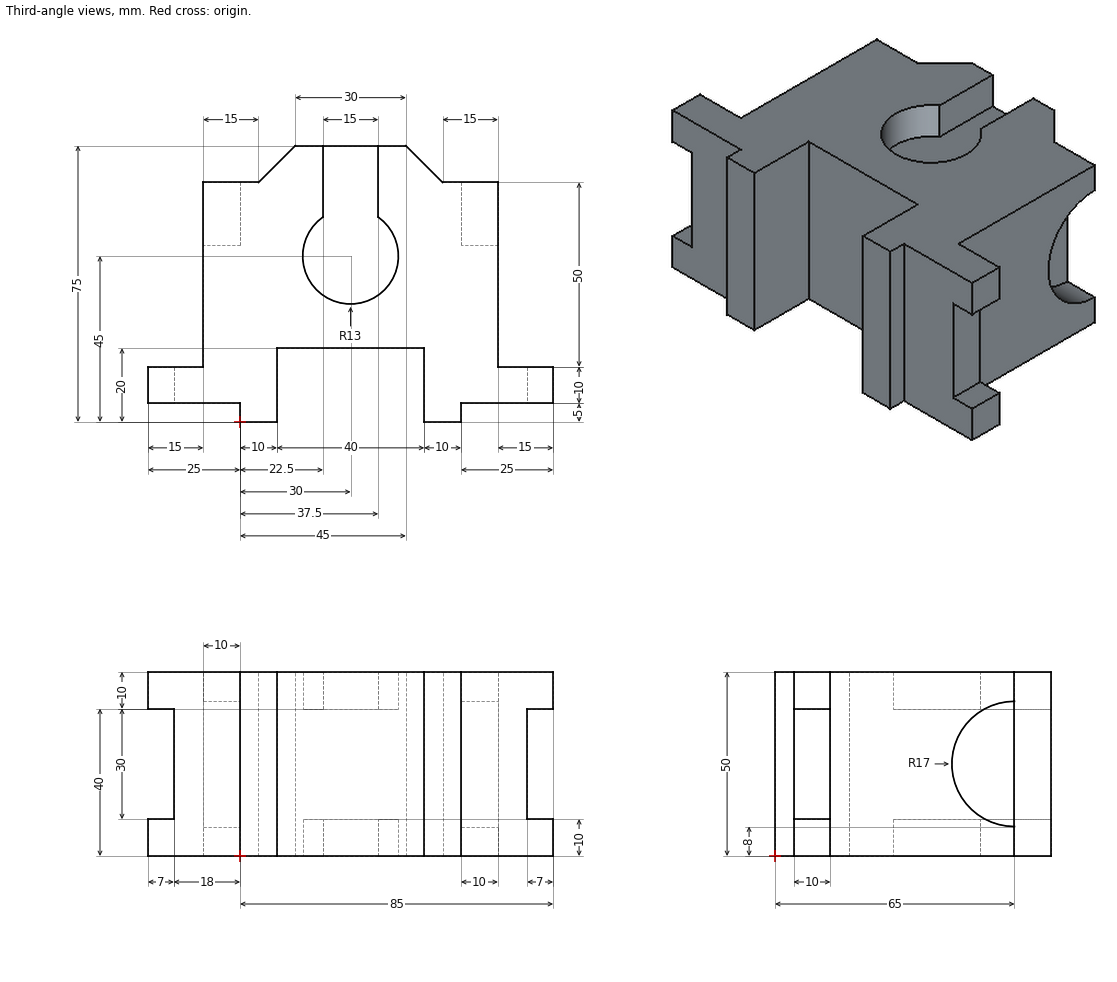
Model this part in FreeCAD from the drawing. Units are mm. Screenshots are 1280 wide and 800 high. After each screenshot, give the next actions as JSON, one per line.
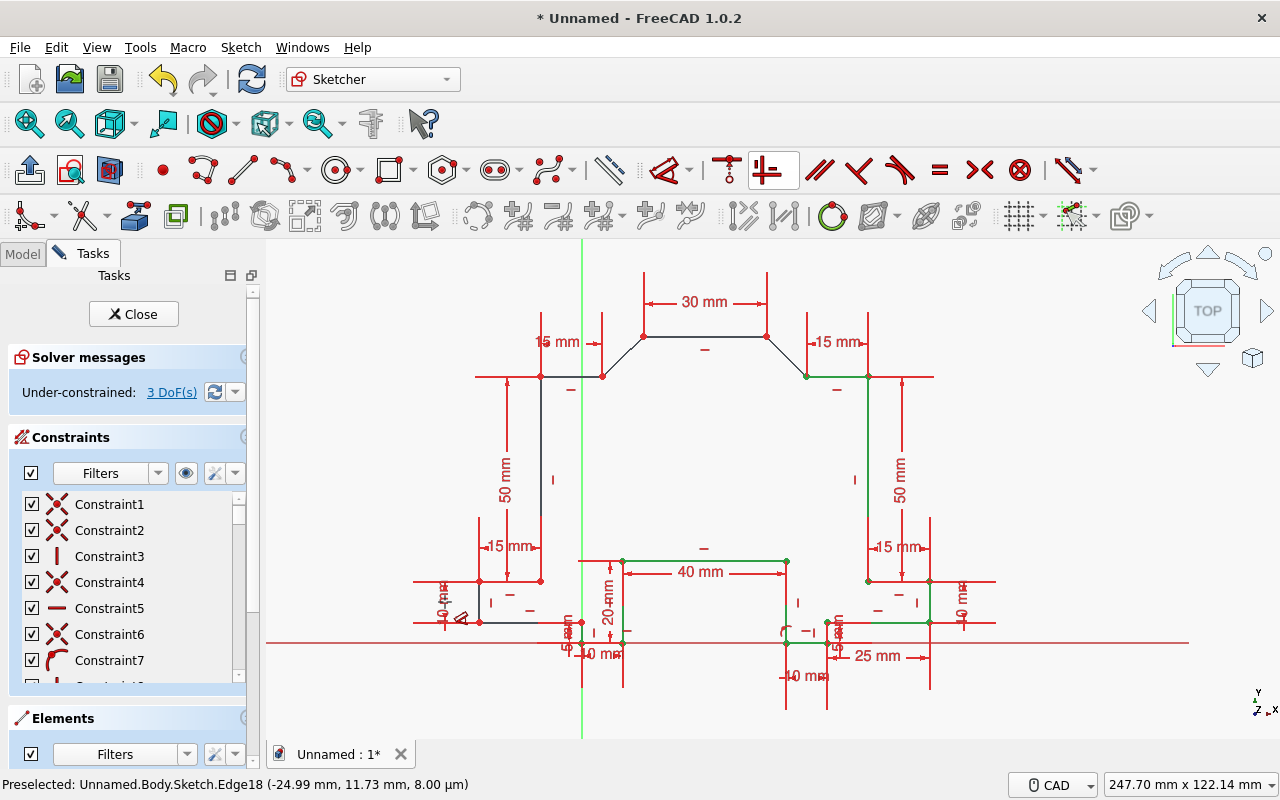
{"action": "left_click", "coordinate": [510, 623]}
{"action": "left_click", "coordinate": [531, 657]}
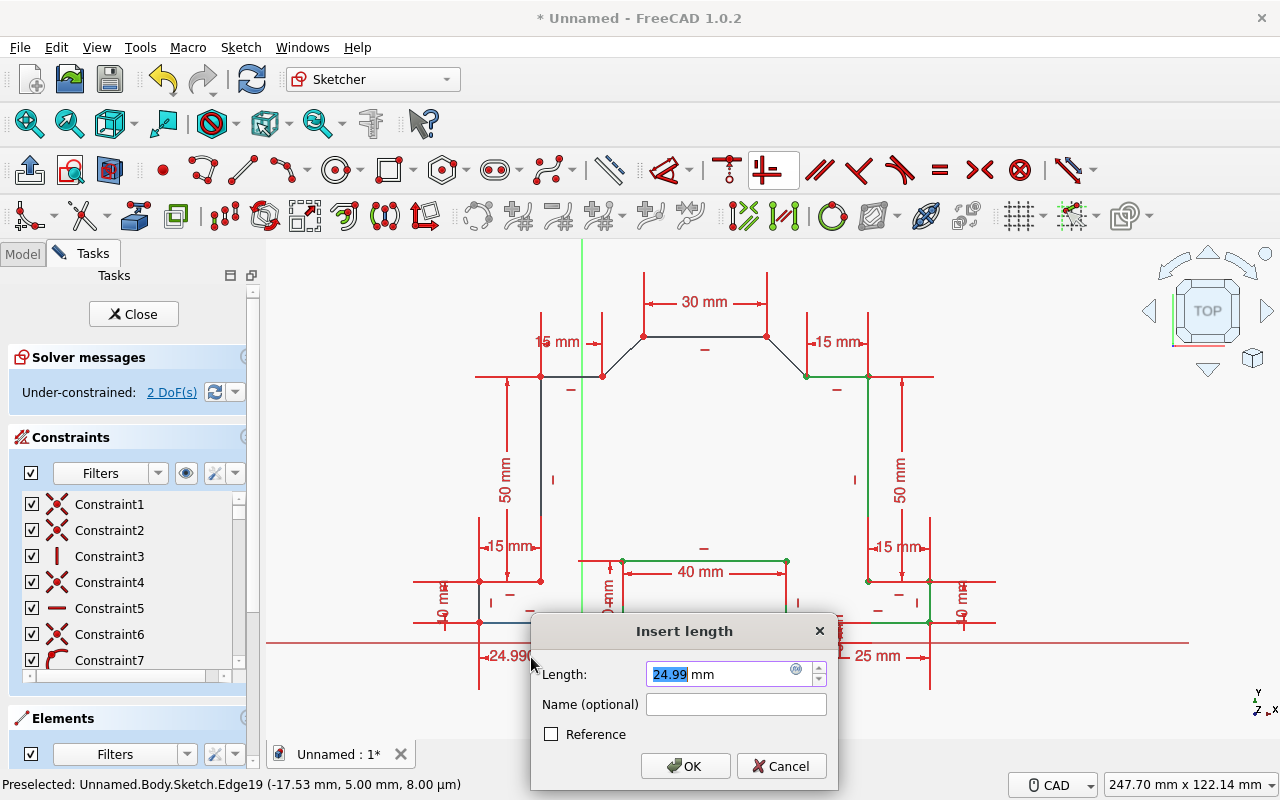
{"action": "type", "text": "25"}
{"action": "key", "text": "Return"}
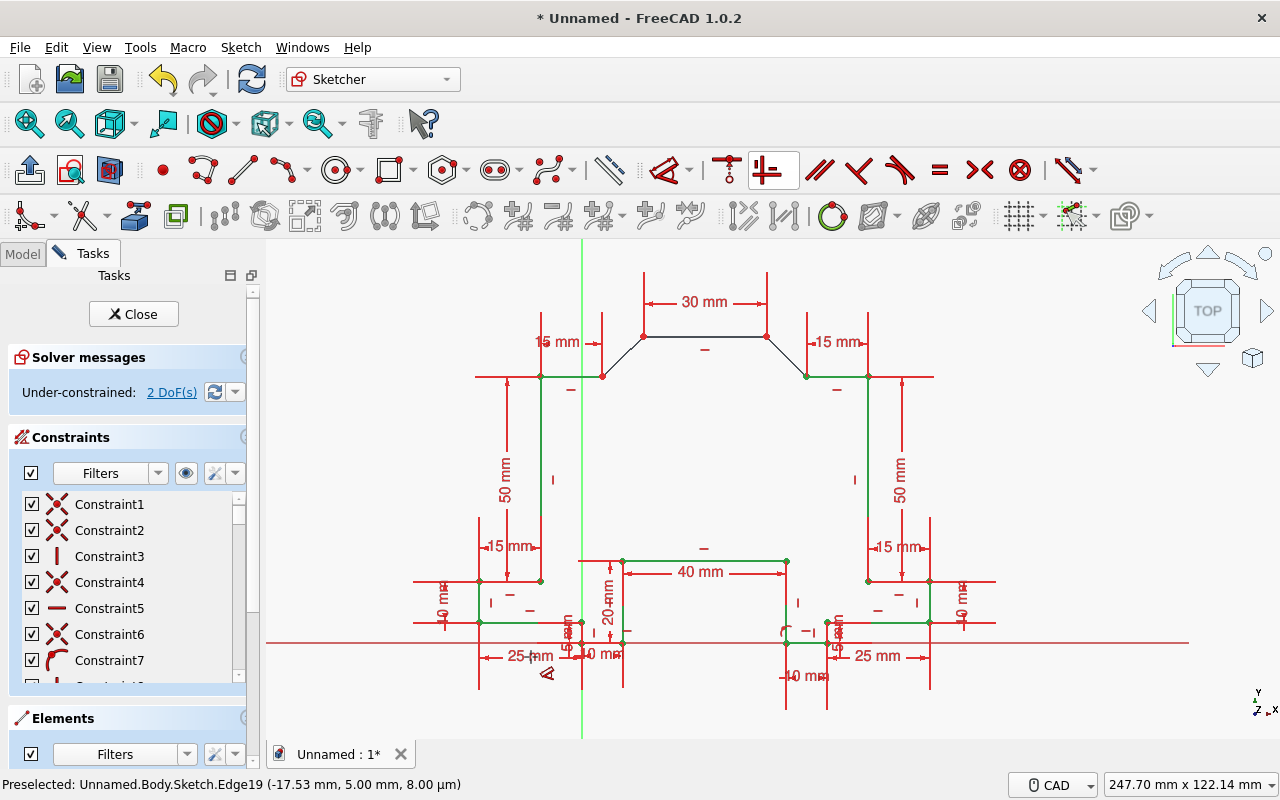
{"action": "left_click", "coordinate": [767, 337]}
{"action": "left_click", "coordinate": [674, 677]}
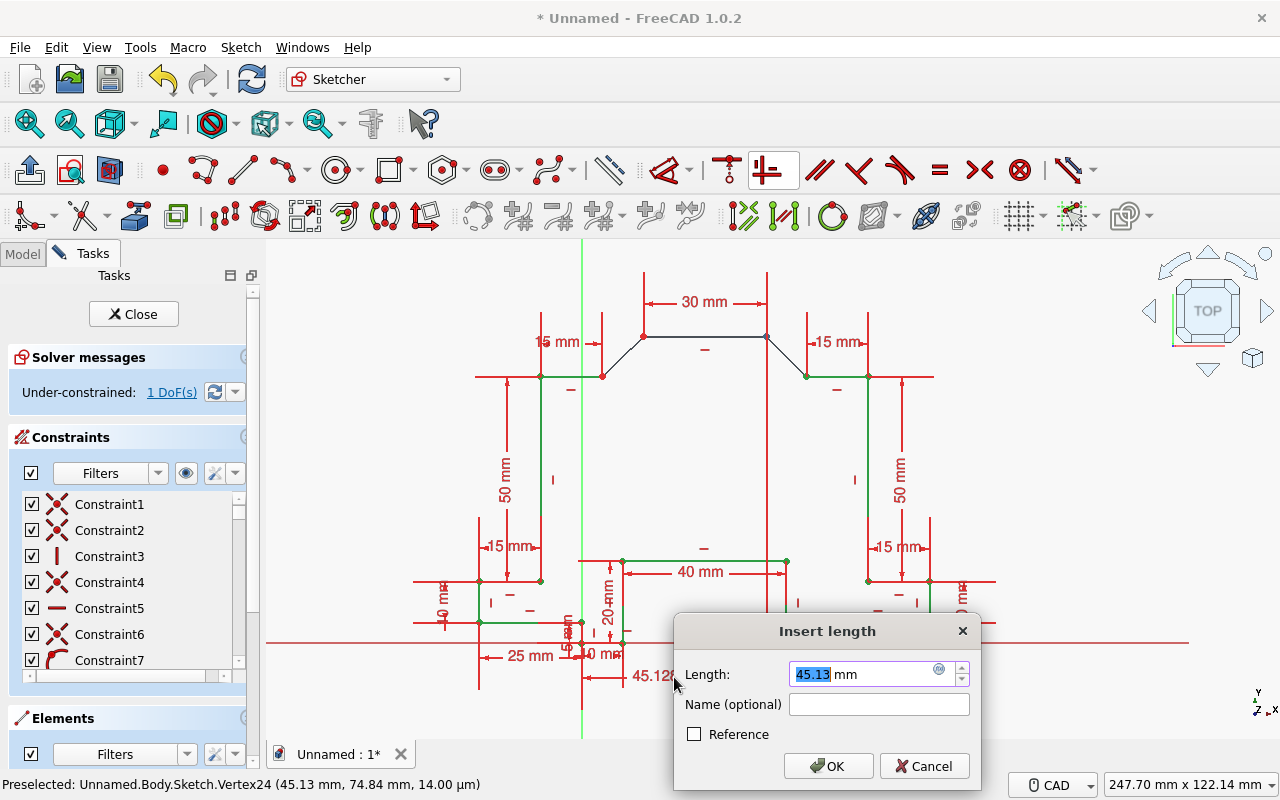
{"action": "type", "text": "45"}
{"action": "key", "text": "Return"}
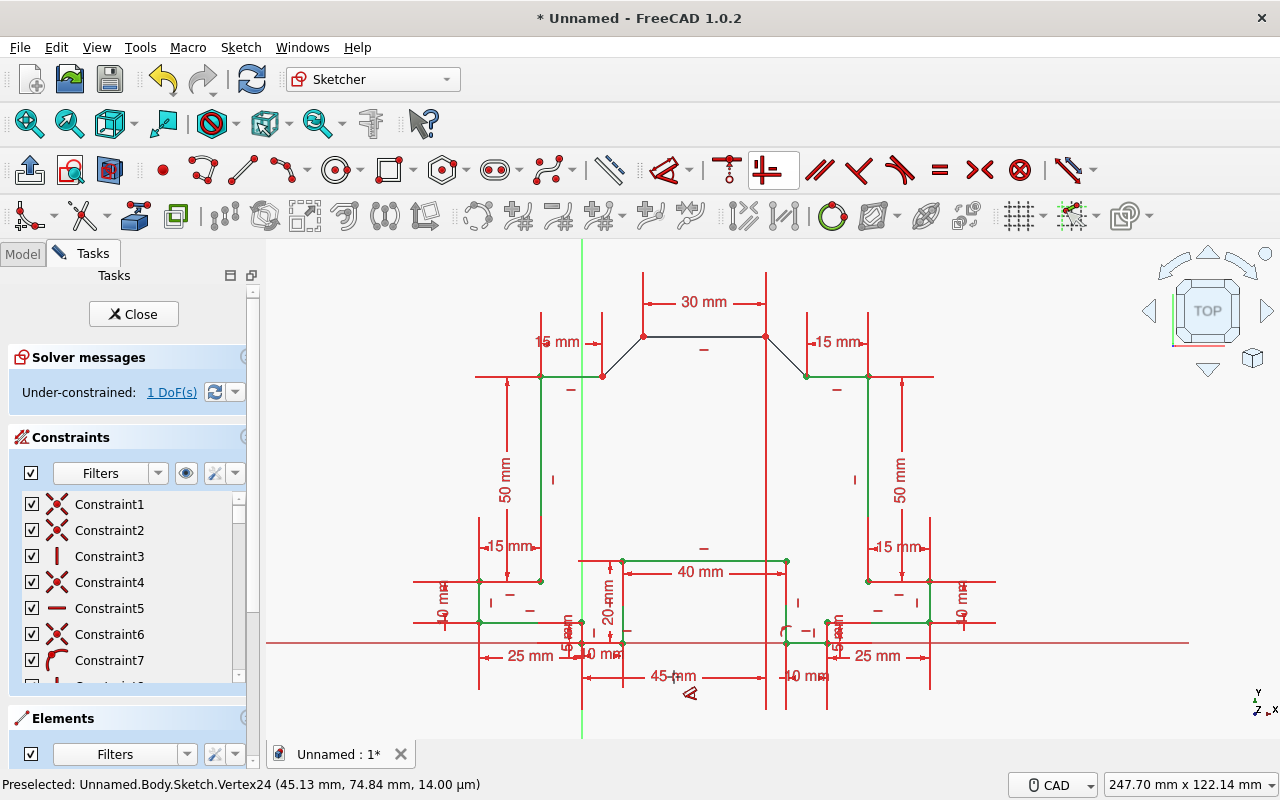
{"action": "left_click", "coordinate": [766, 337]}
{"action": "left_click", "coordinate": [800, 490]}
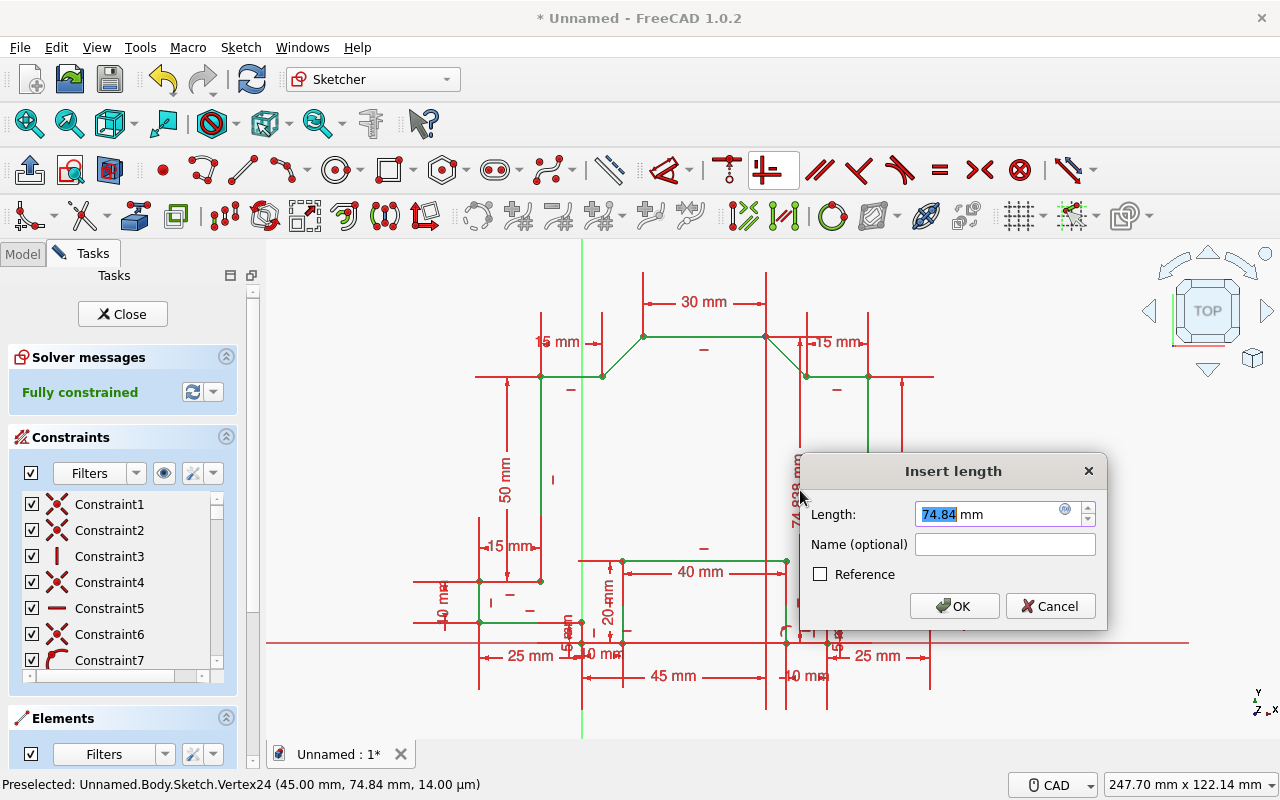
{"action": "type", "text": "75"}
{"action": "key", "text": "Return"}
{"action": "key", "text": "Escape"}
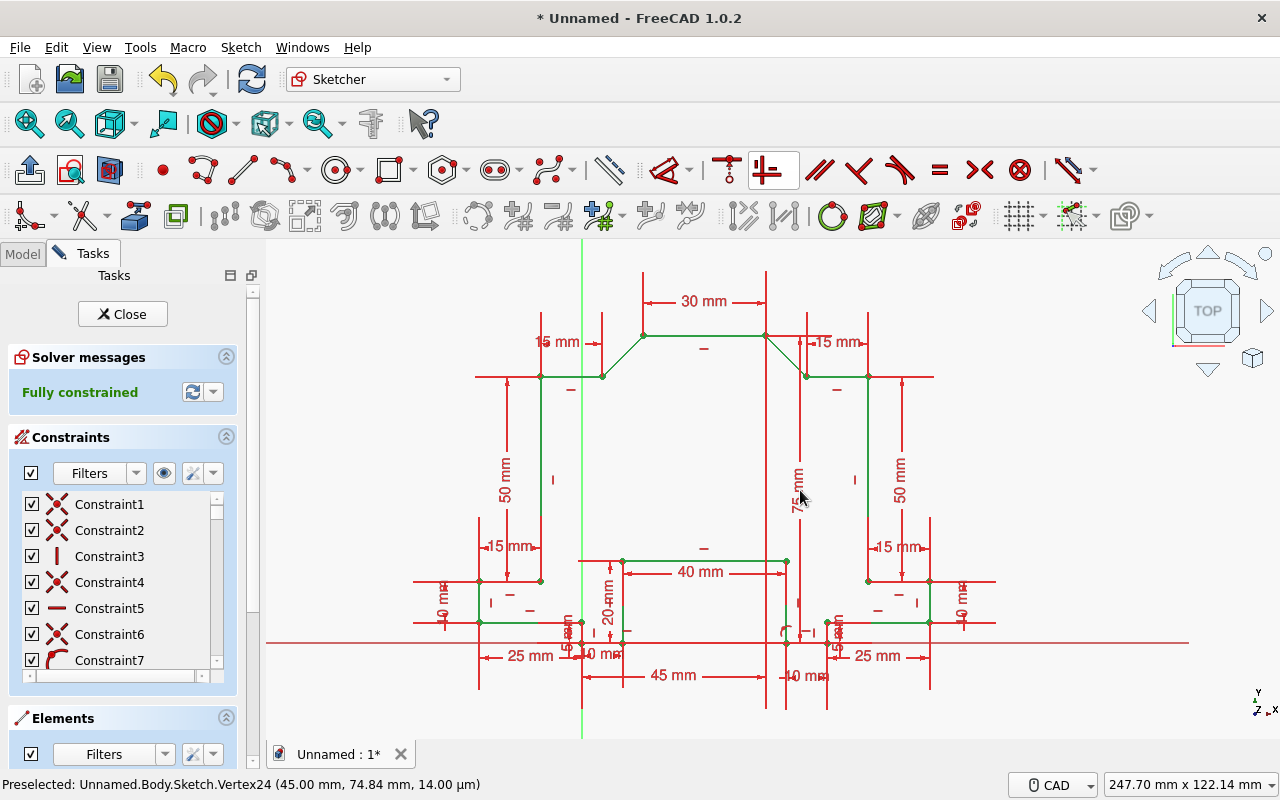
{"action": "left_click", "coordinate": [123, 314]}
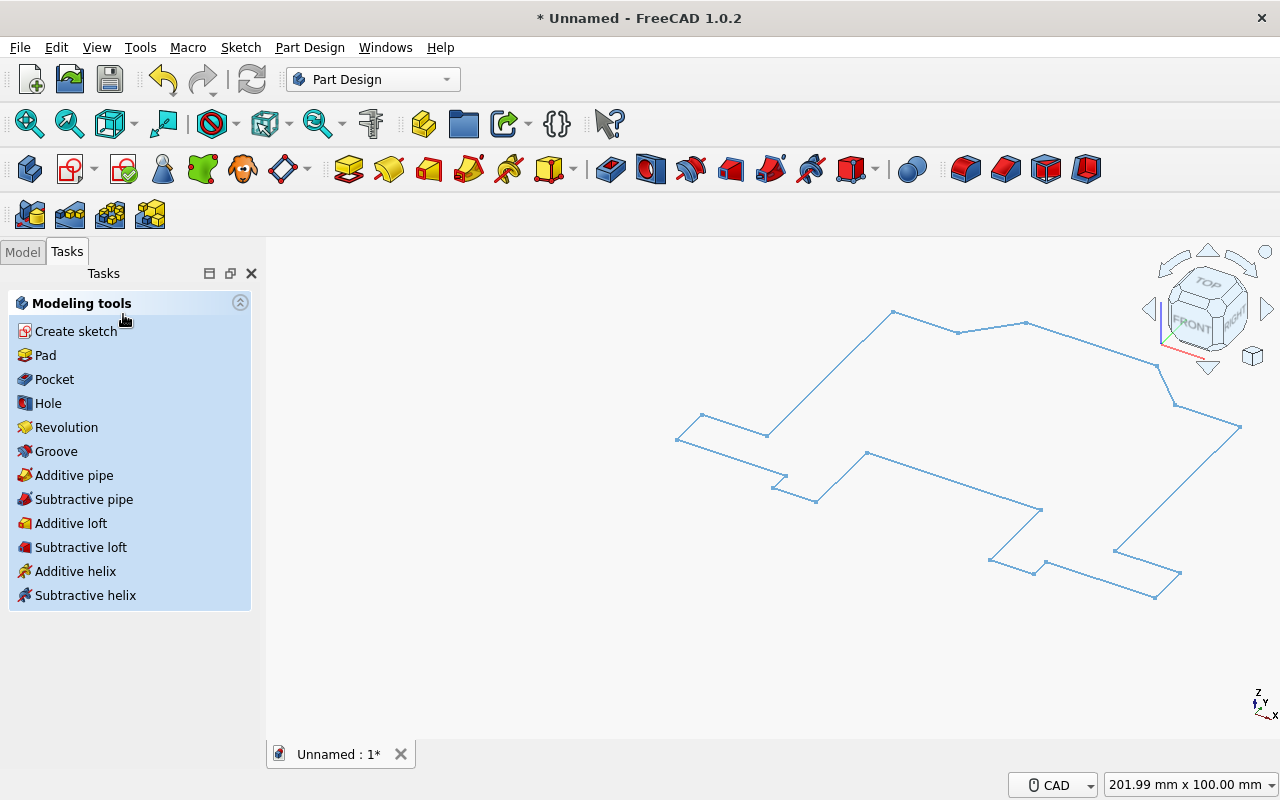
{"action": "left_click", "coordinate": [350, 170]}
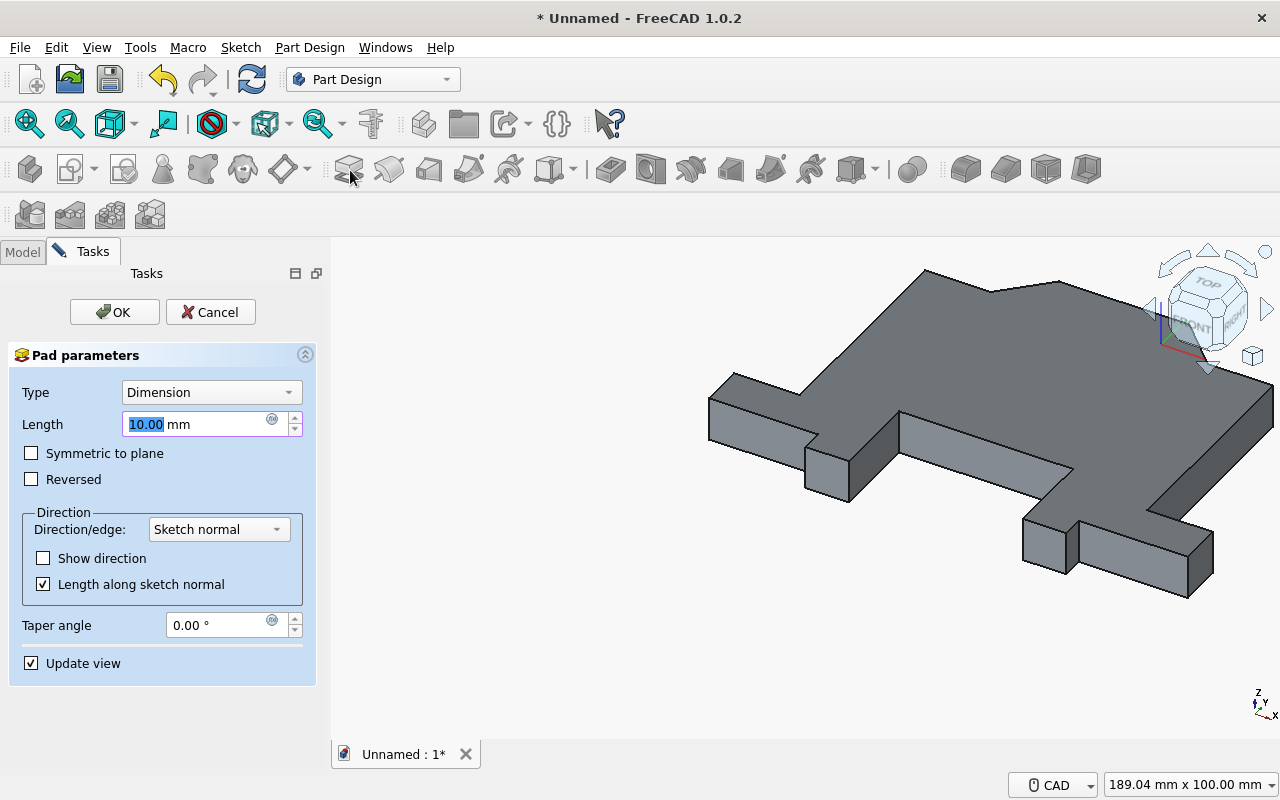
{"action": "type", "text": "50"}
{"action": "key", "text": "Tab"}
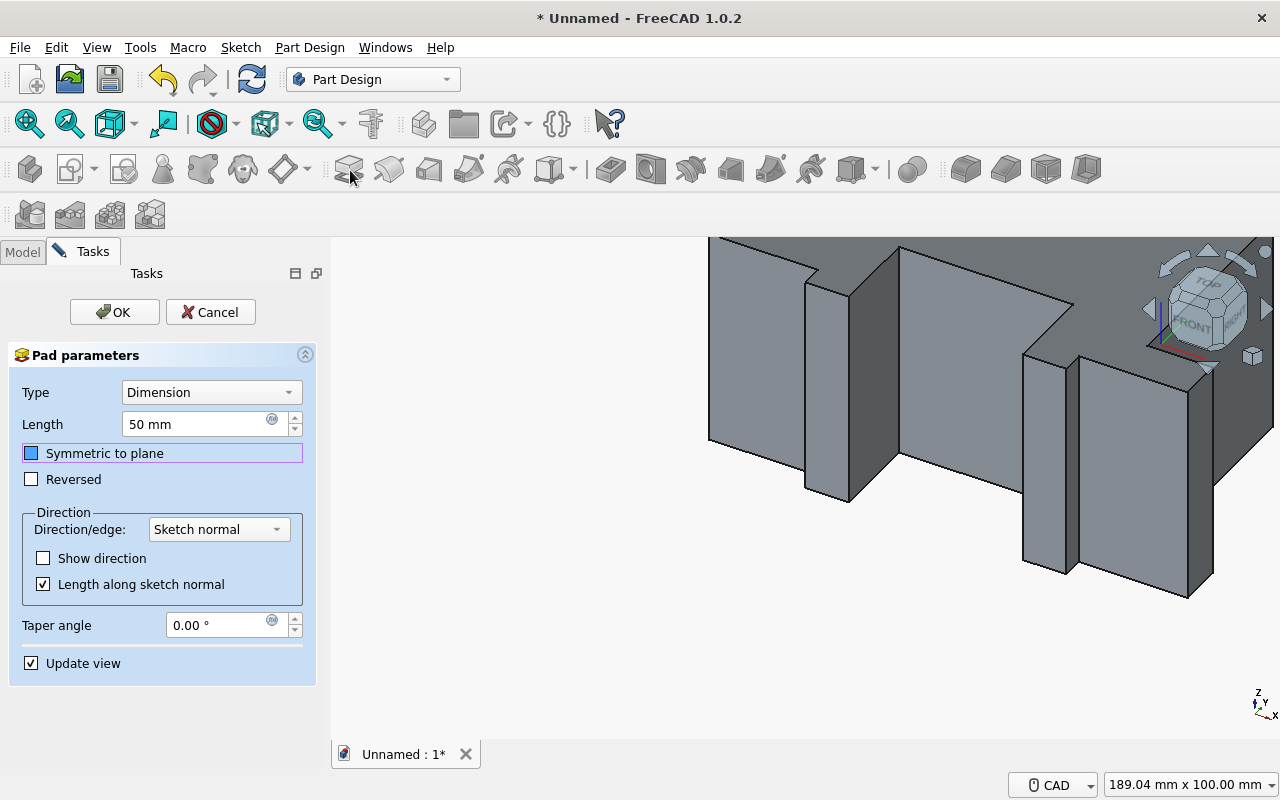
{"action": "left_click", "coordinate": [115, 312]}